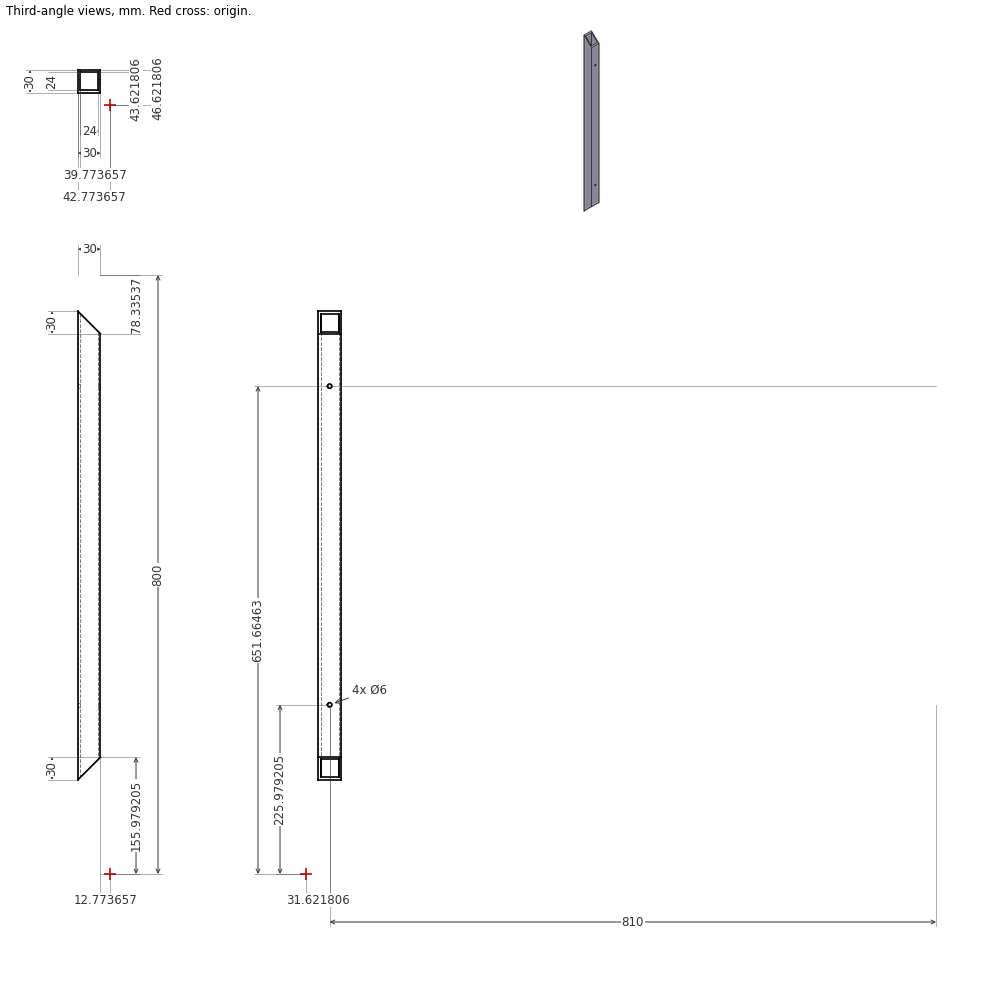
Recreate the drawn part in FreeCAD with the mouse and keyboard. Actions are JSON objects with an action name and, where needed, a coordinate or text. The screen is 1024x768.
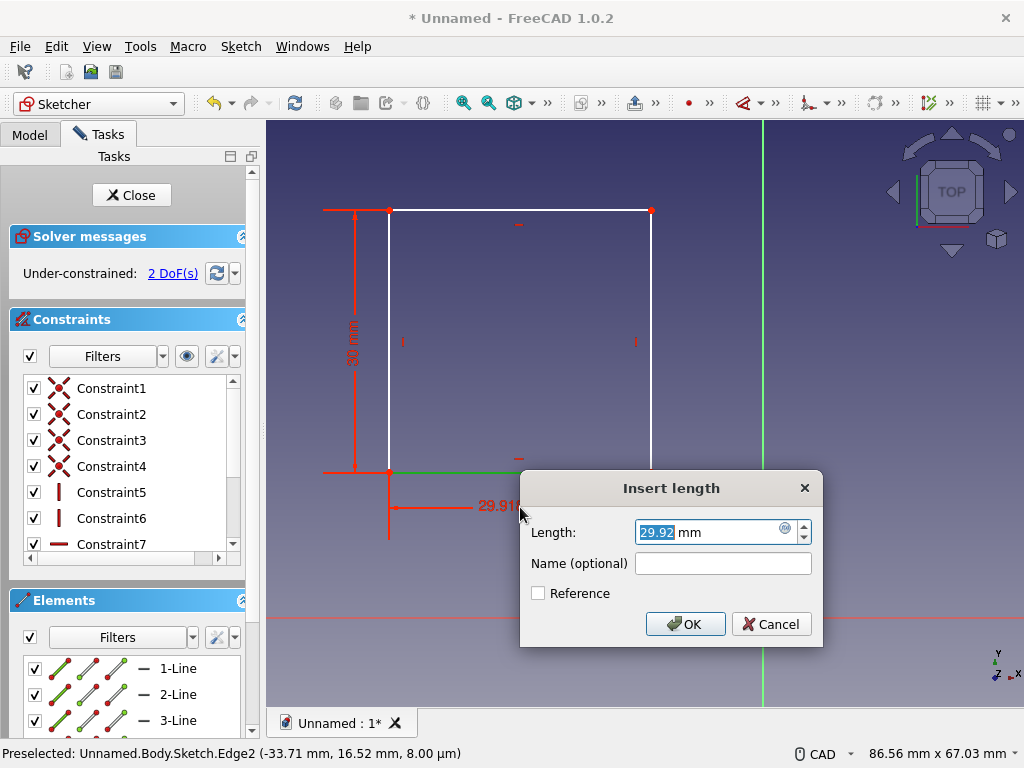
{"action": "type", "text": "30"}
{"action": "key", "text": "Return"}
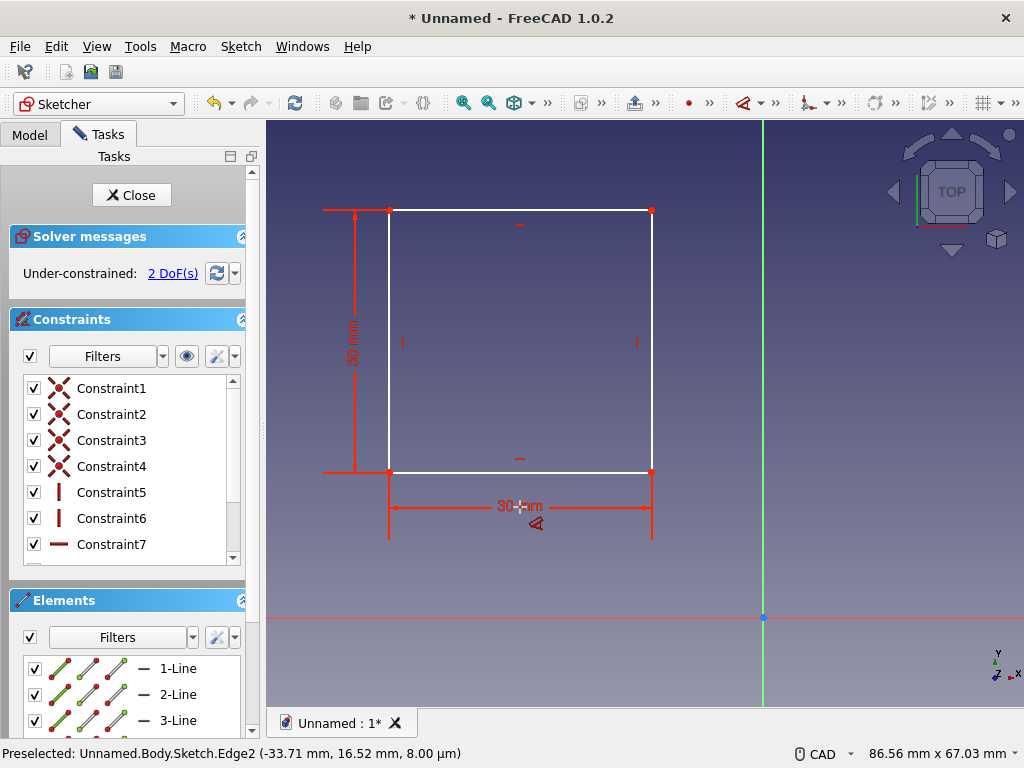
{"action": "left_click", "coordinate": [389, 210]}
{"action": "left_click", "coordinate": [576, 652]}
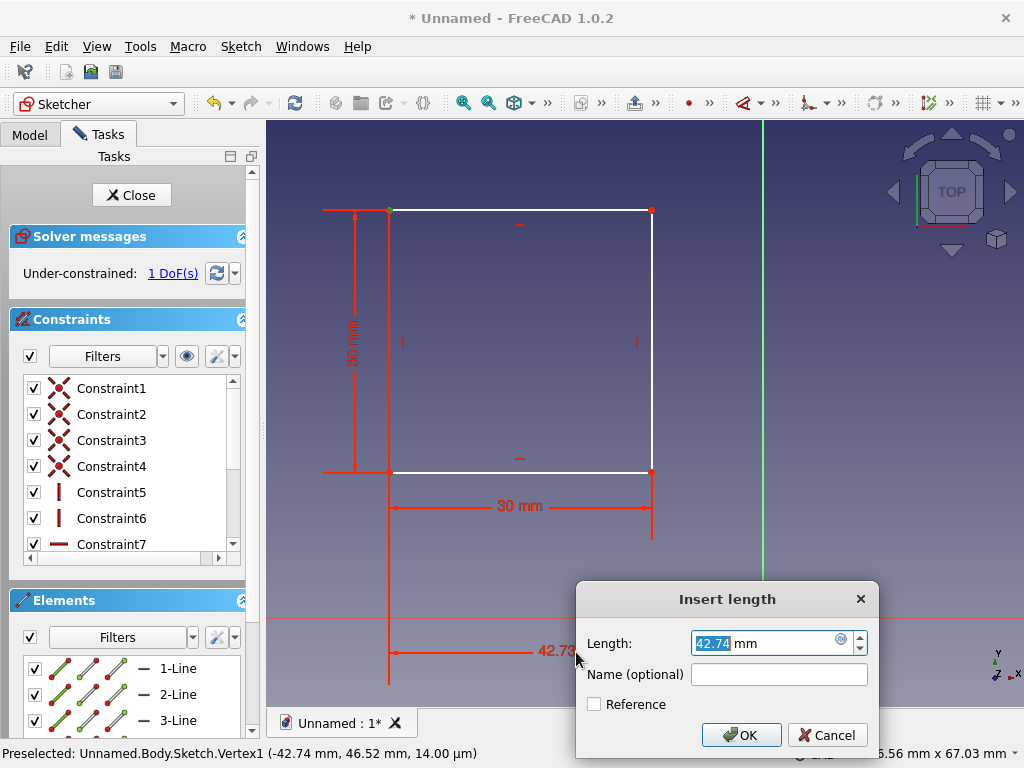
{"action": "type", "text": "42.773657"}
{"action": "key", "text": "Return"}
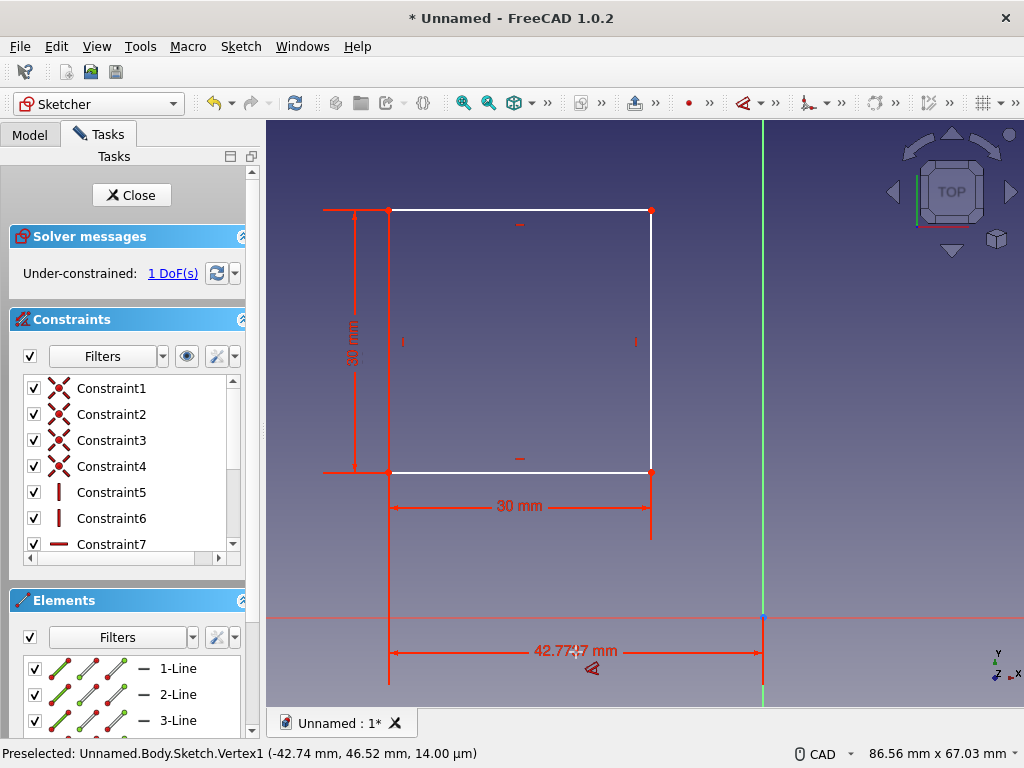
{"action": "left_click", "coordinate": [389, 210]}
{"action": "left_click", "coordinate": [355, 414]}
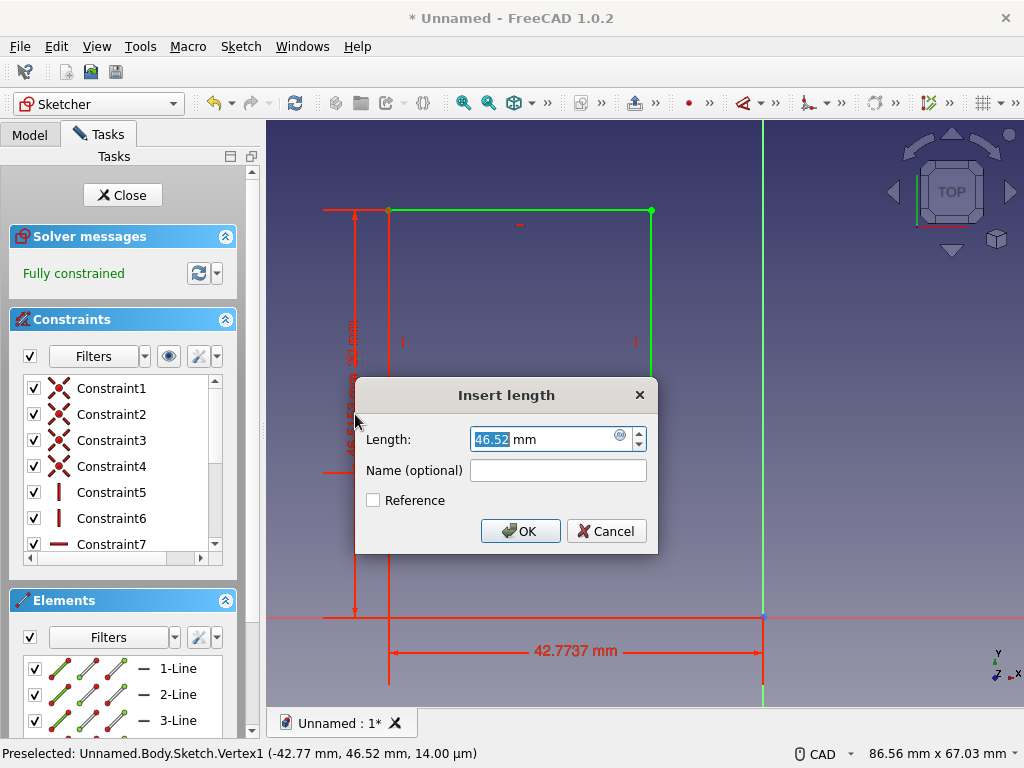
{"action": "type", "text": "46.621806"}
{"action": "key", "text": "Return"}
{"action": "key", "text": "Escape"}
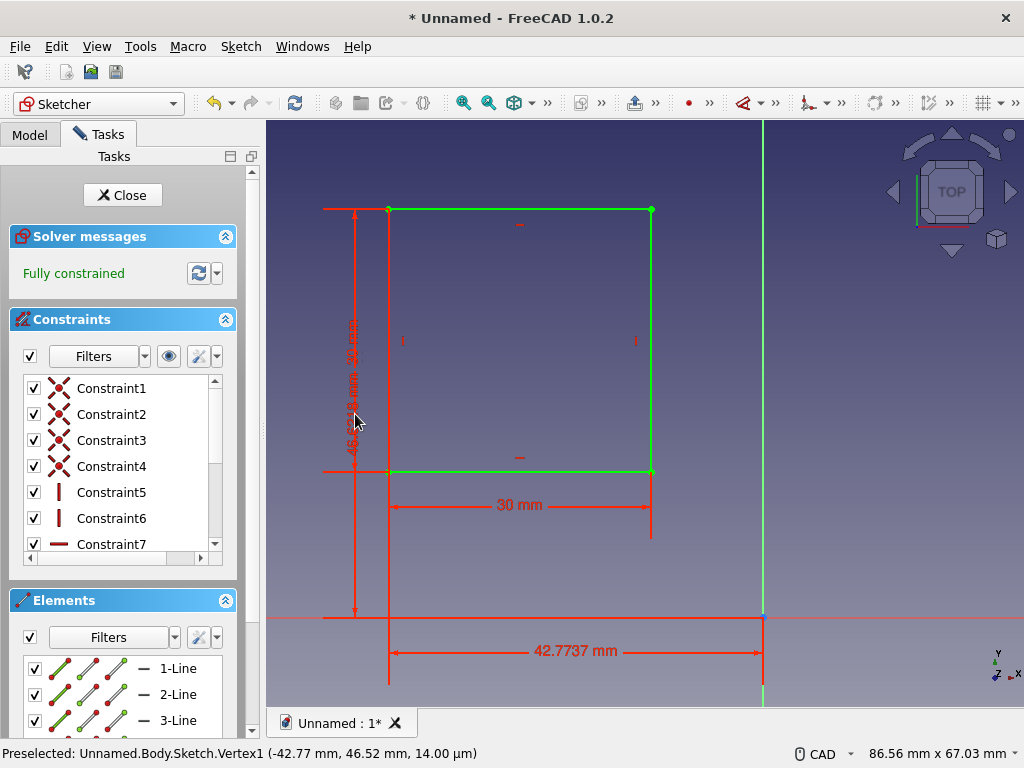
{"action": "left_click", "coordinate": [123, 195]}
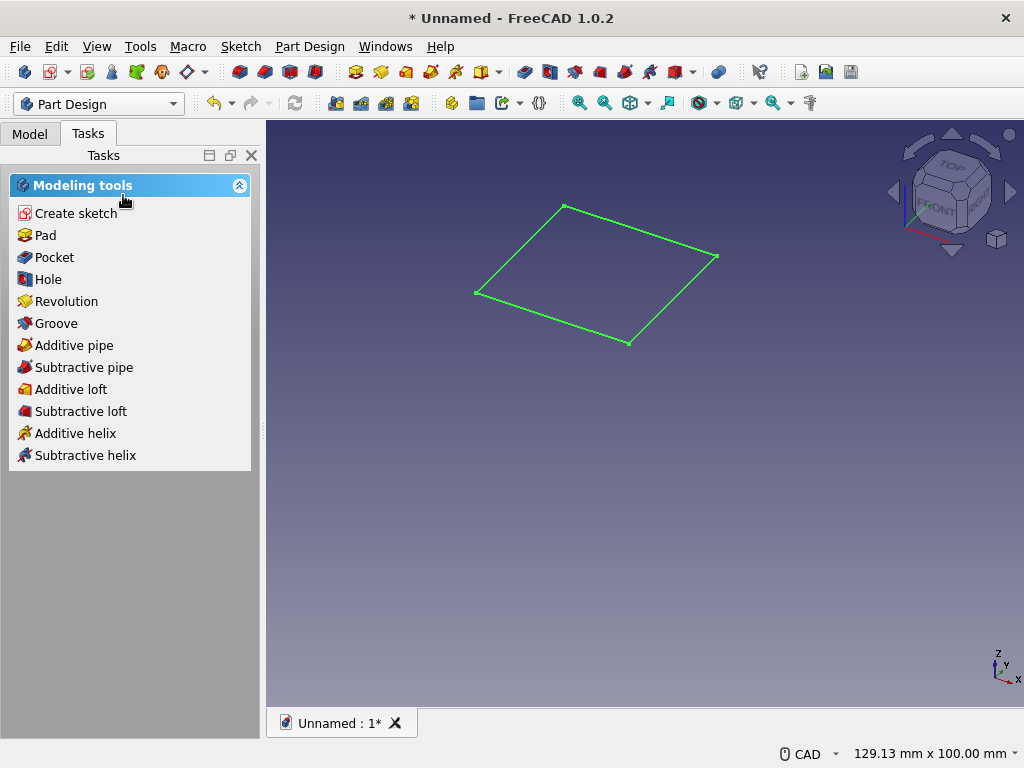
{"action": "left_click", "coordinate": [356, 72]}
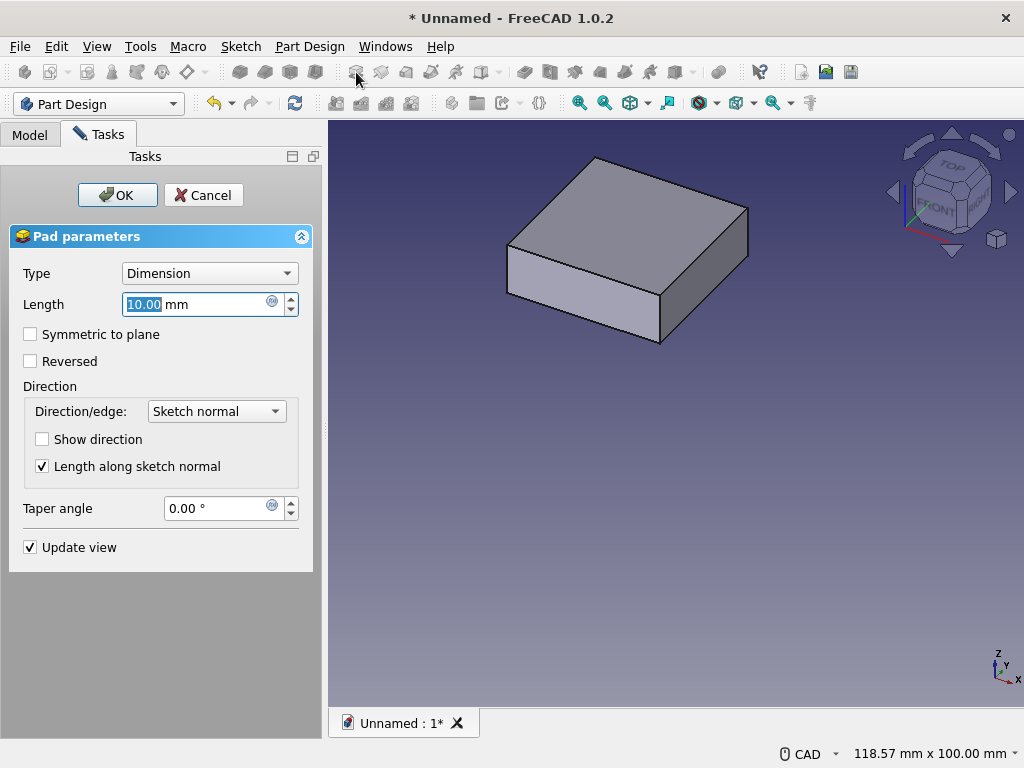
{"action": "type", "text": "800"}
{"action": "key", "text": "Tab"}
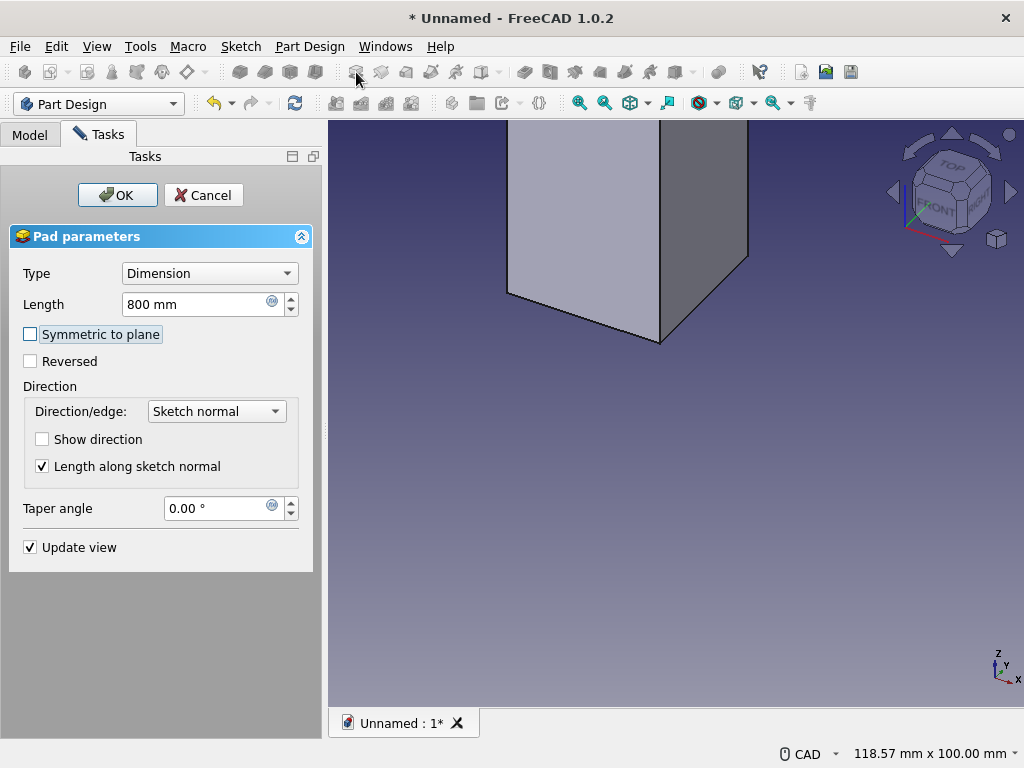
{"action": "left_click", "coordinate": [118, 195]}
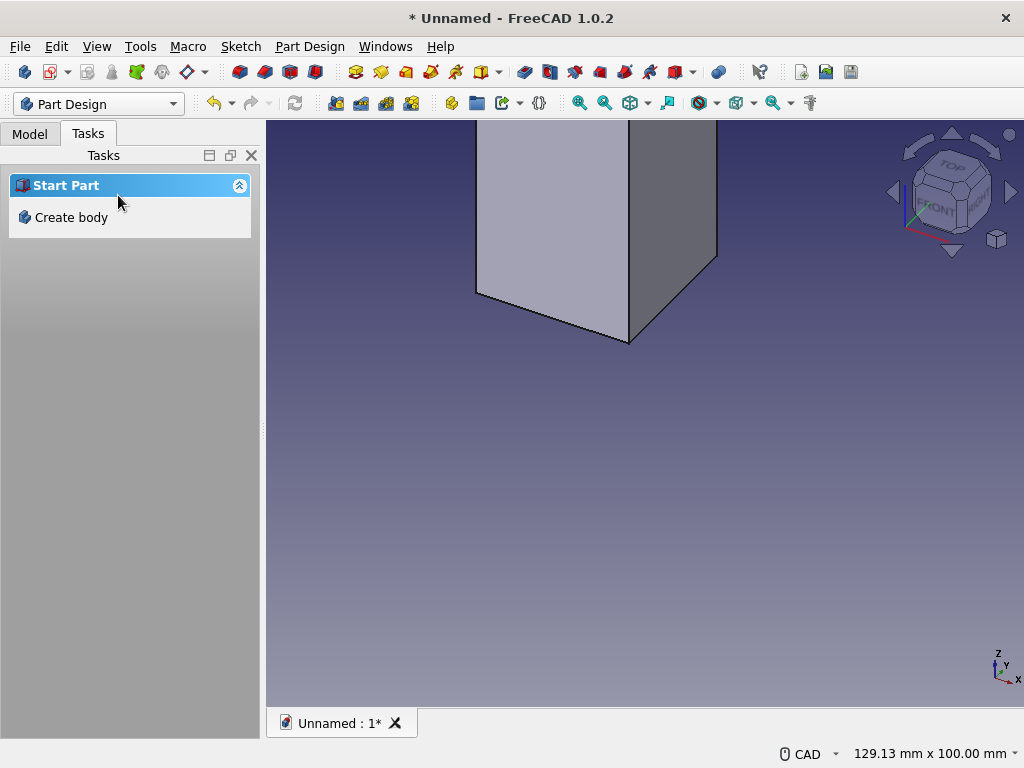
{"action": "left_click", "coordinate": [580, 104]}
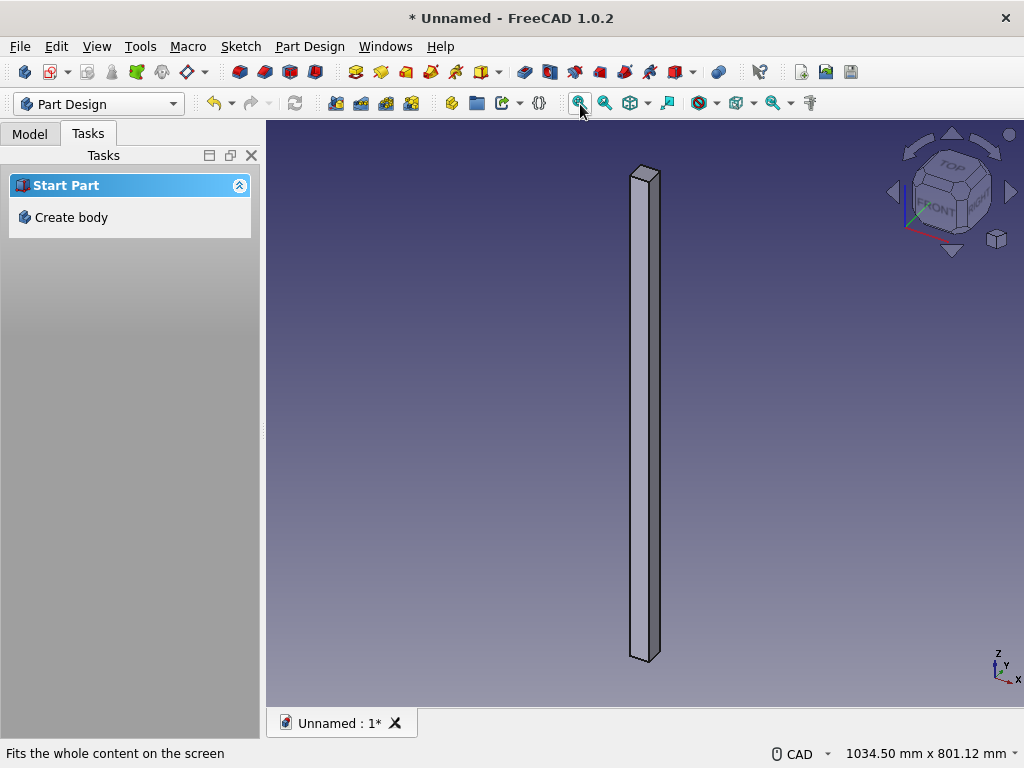
{"action": "left_click", "coordinate": [644, 170]}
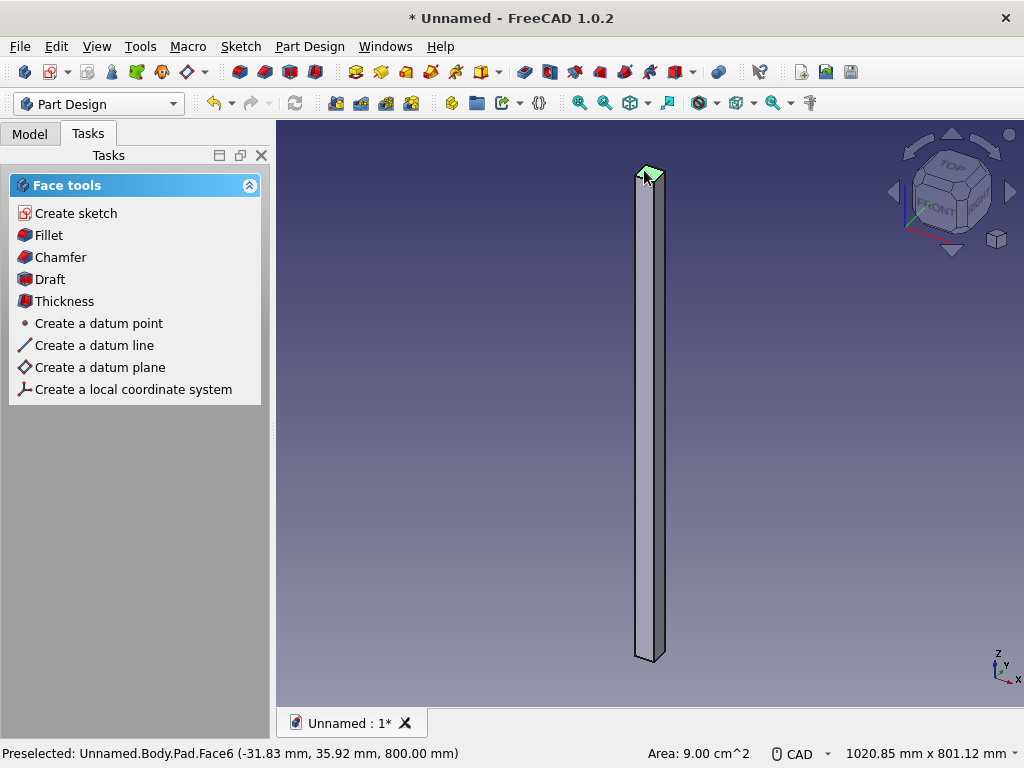
{"action": "left_click", "coordinate": [50, 72]}